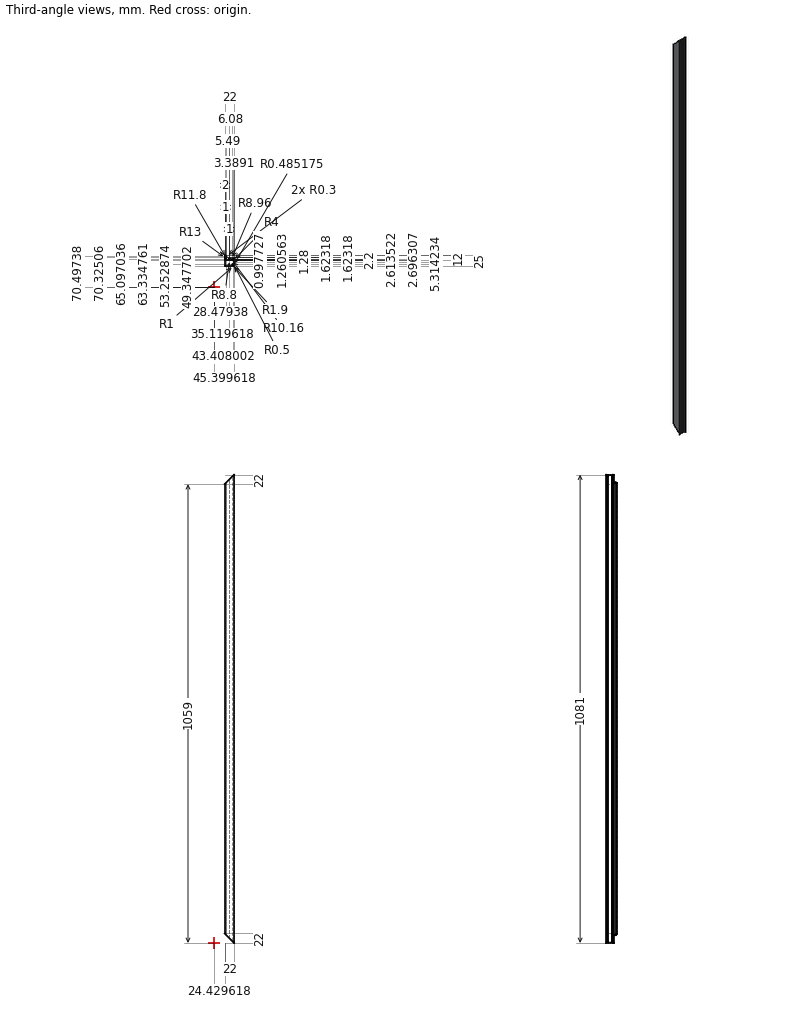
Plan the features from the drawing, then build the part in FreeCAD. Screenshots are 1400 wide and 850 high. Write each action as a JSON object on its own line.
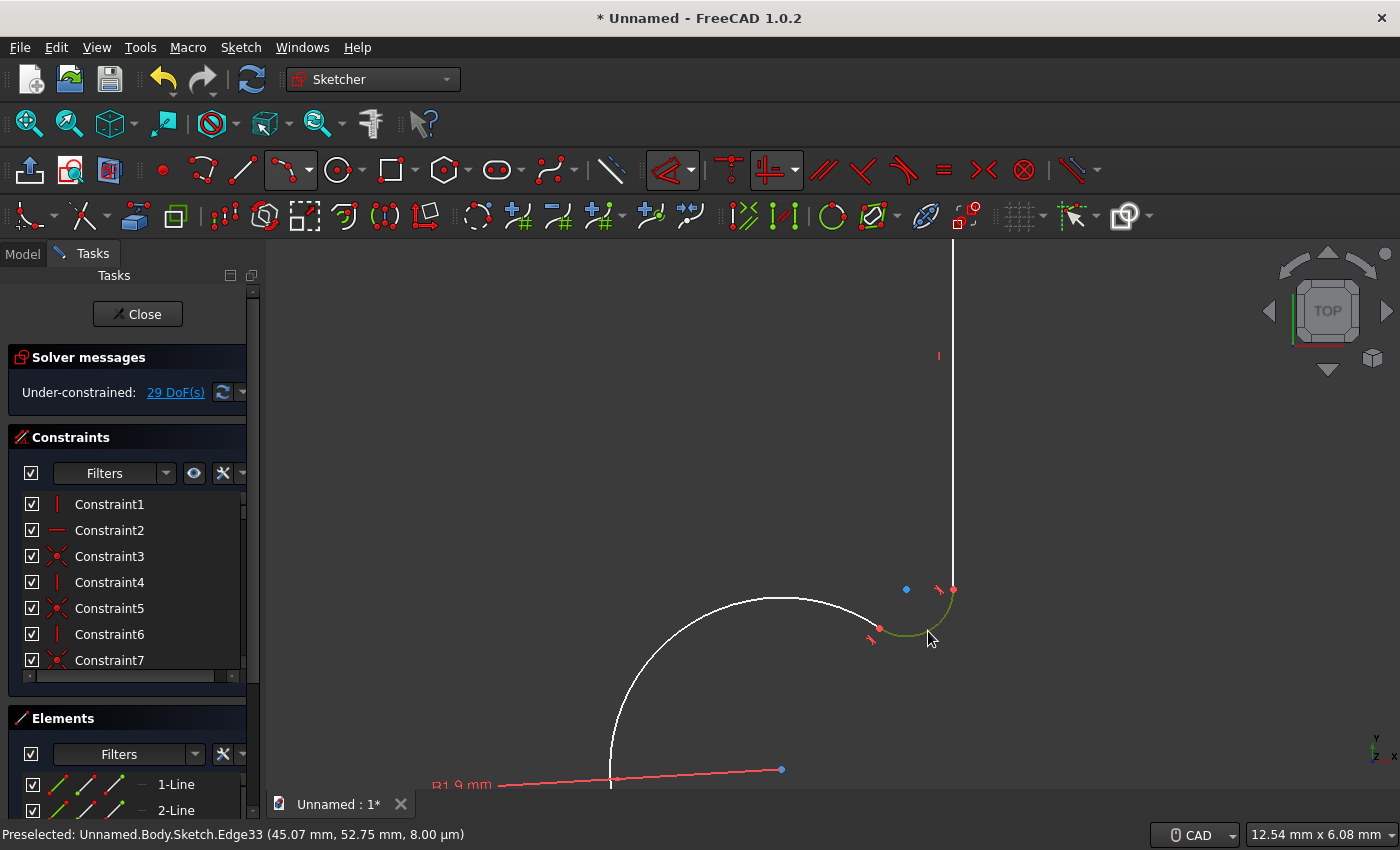
{"action": "key", "text": "k r"}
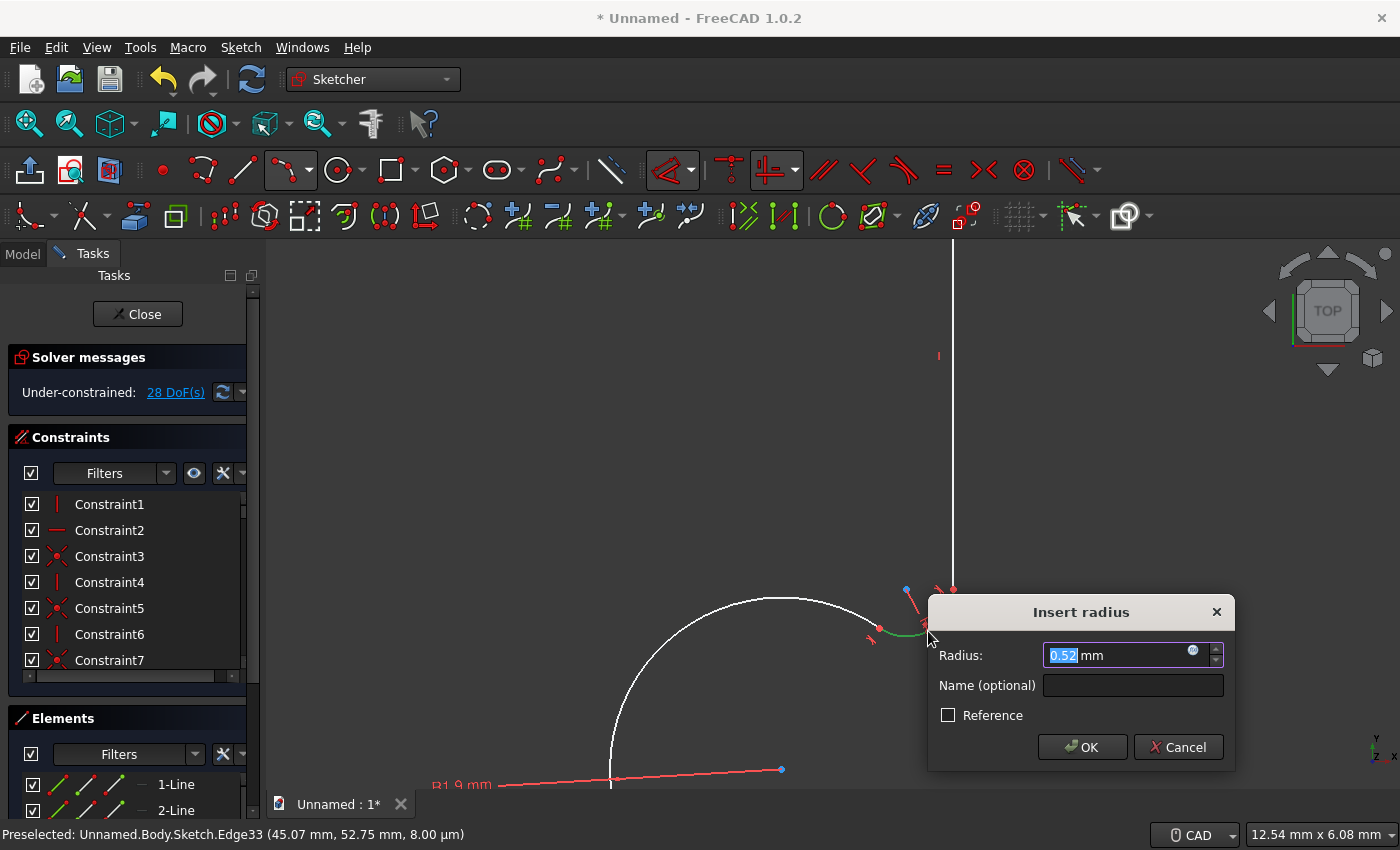
{"action": "type", "text": "0.5"}
{"action": "key", "text": "Return"}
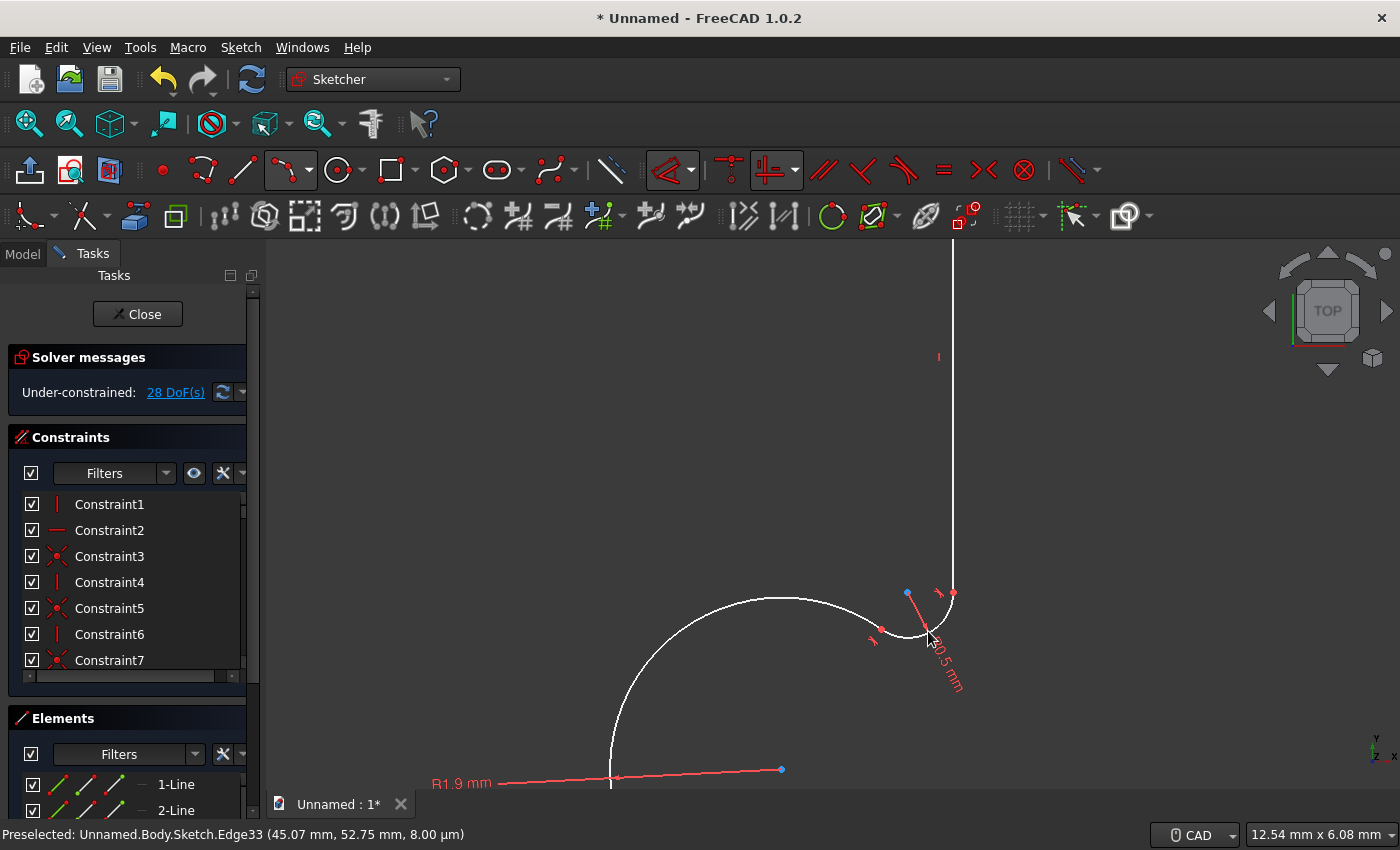
{"action": "scroll", "coordinate": [906, 633], "scroll_direction": "down", "scroll_amount": 9}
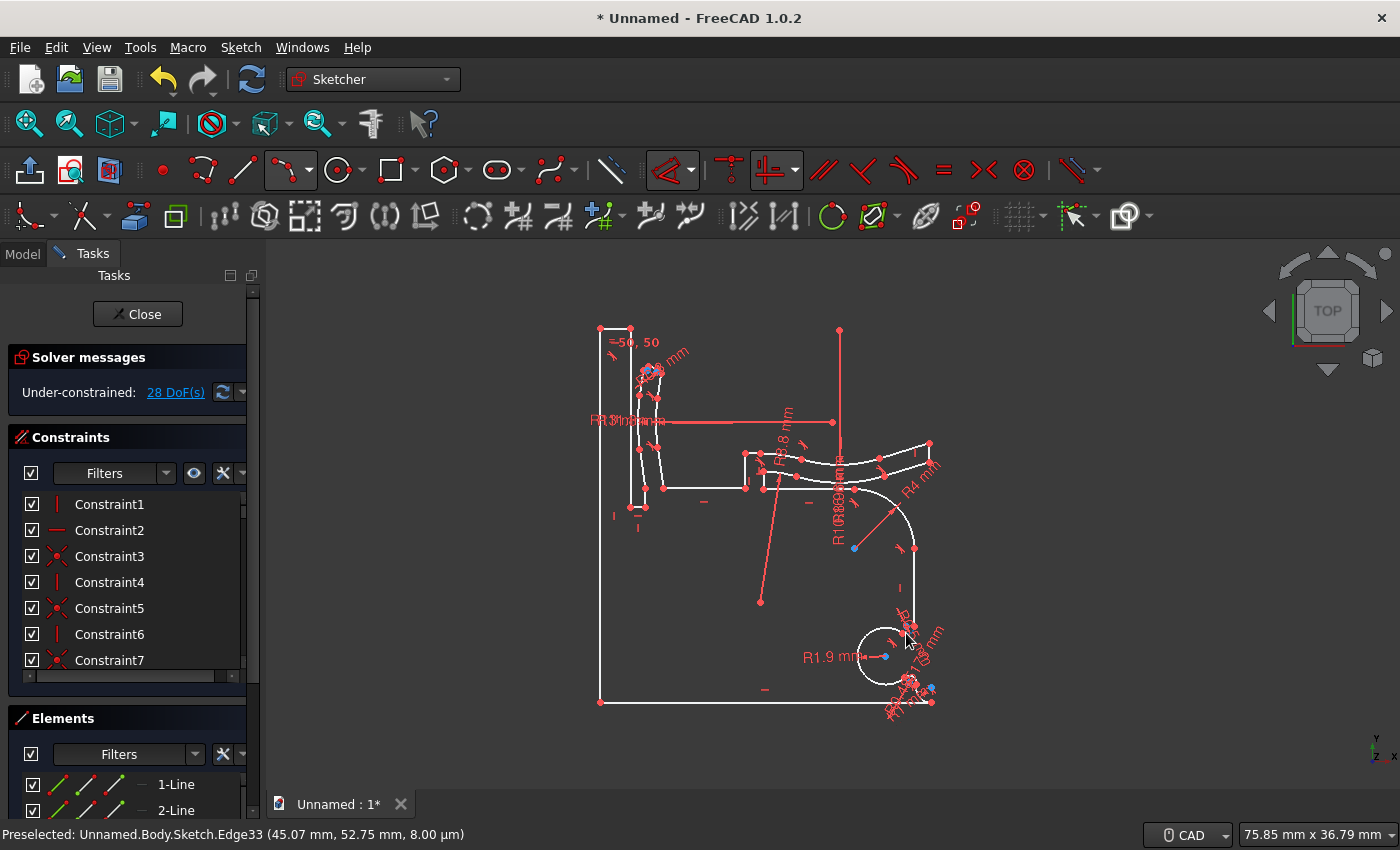
{"action": "scroll", "coordinate": [756, 453], "scroll_direction": "up", "scroll_amount": 6}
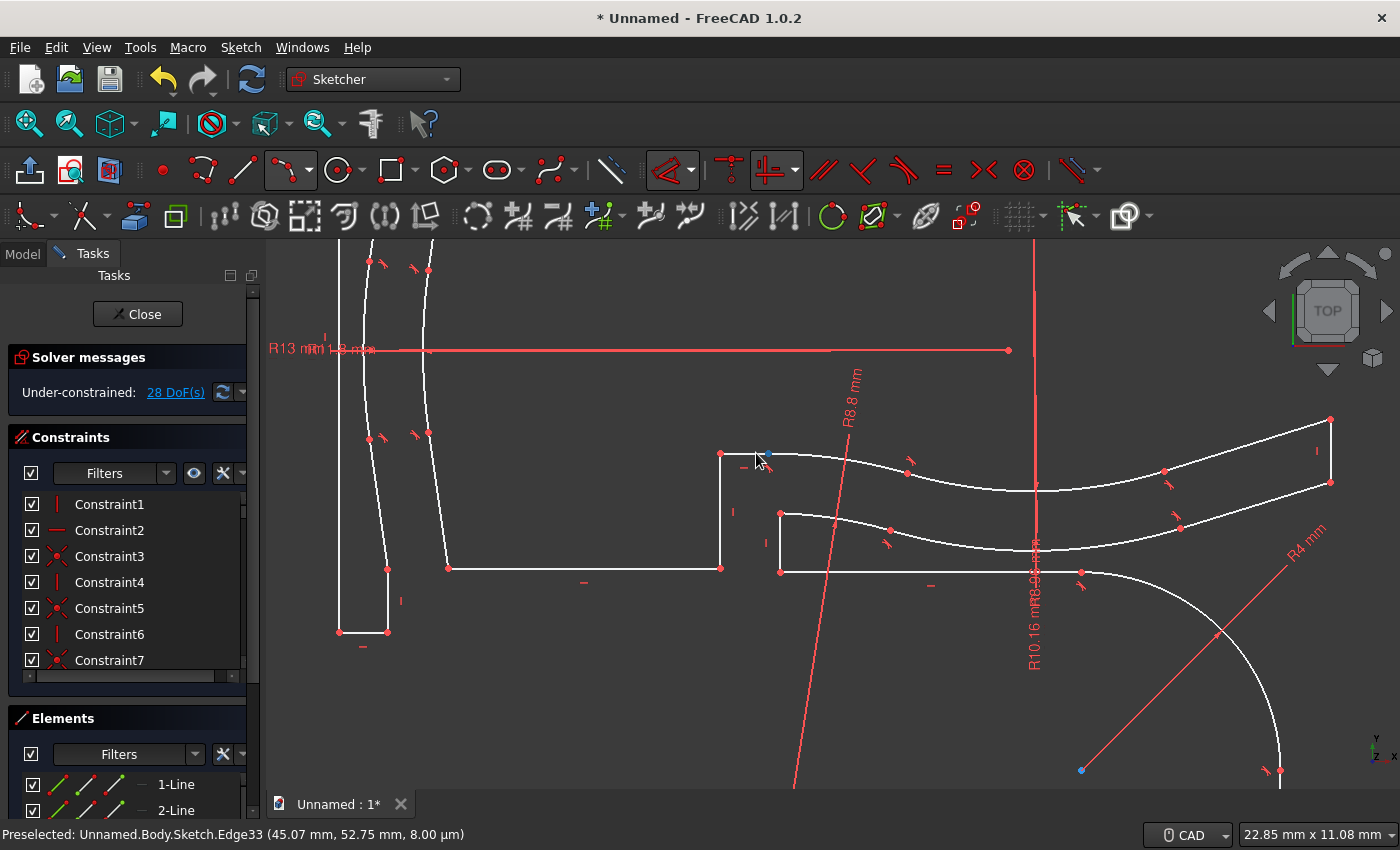
{"action": "left_click", "coordinate": [754, 454]}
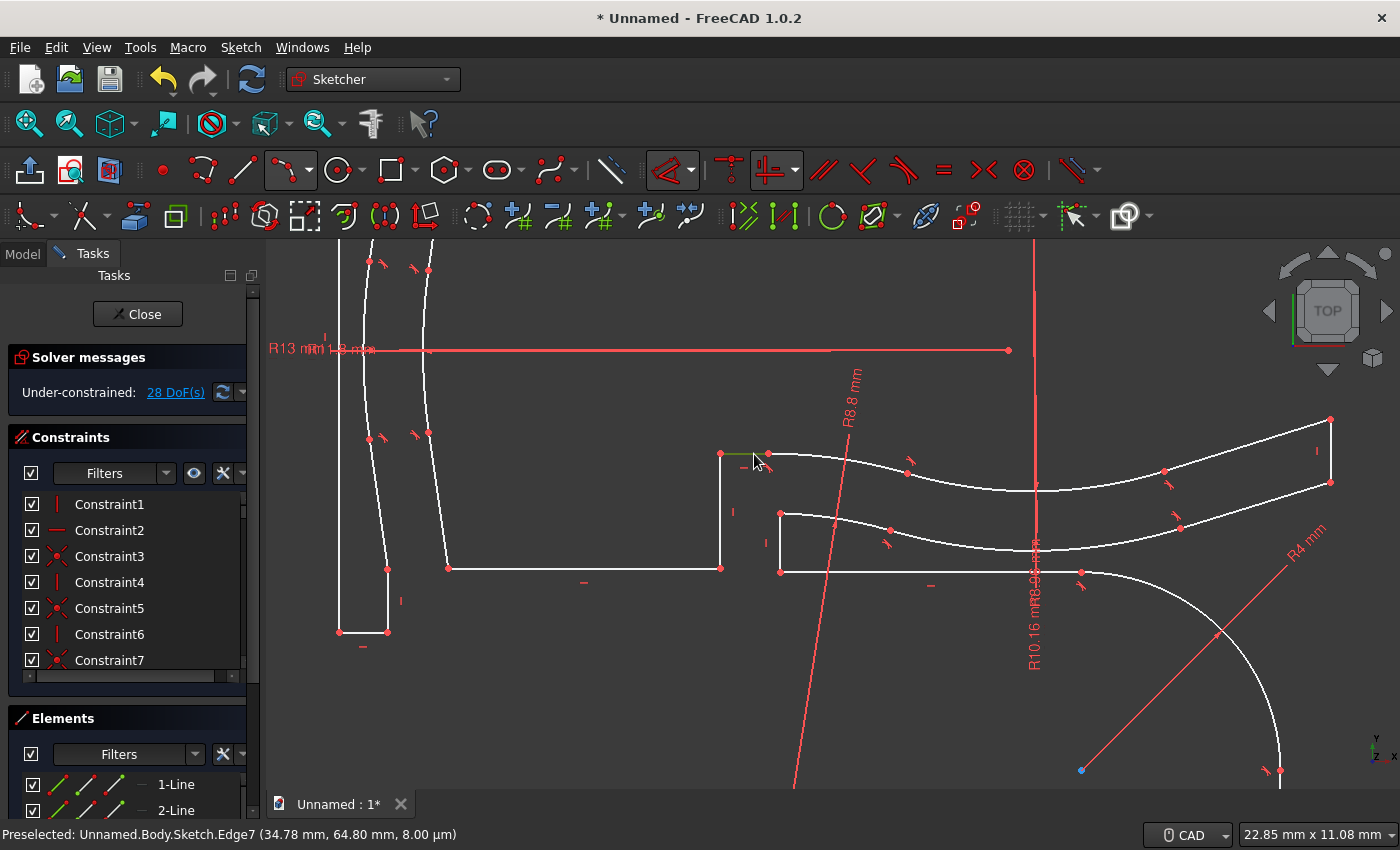
{"action": "left_click", "coordinate": [694, 170]}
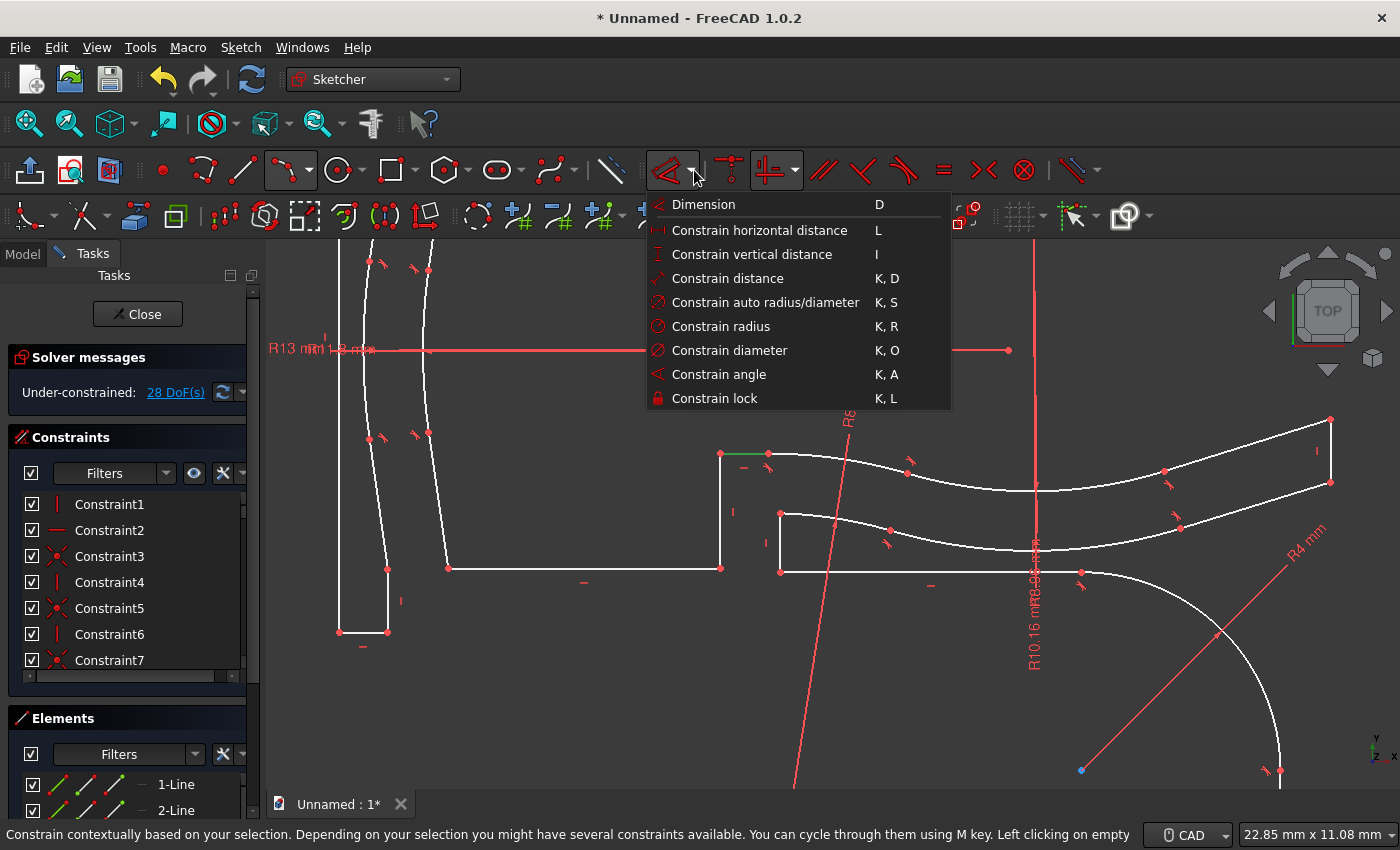
{"action": "left_click", "coordinate": [799, 230]}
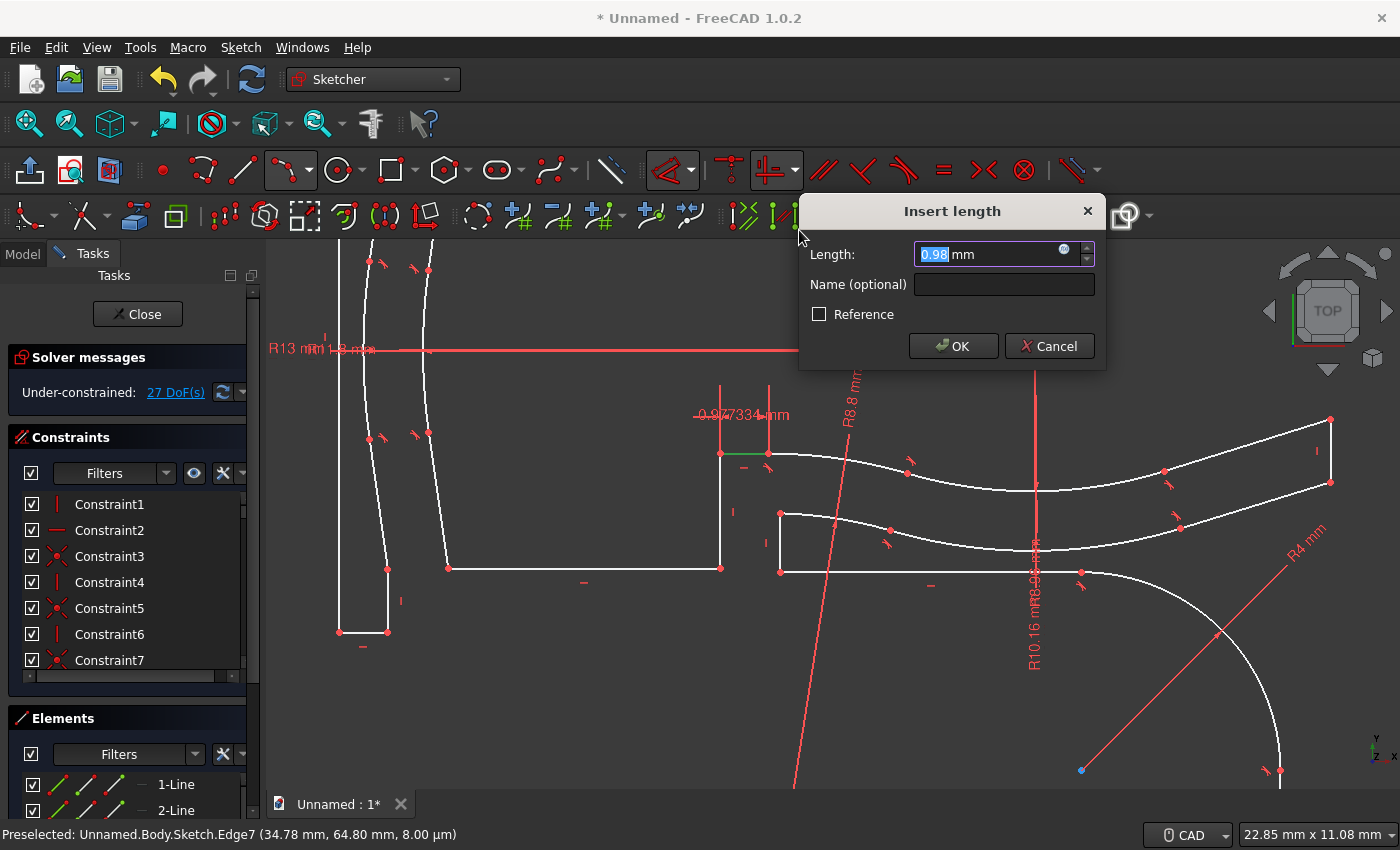
{"action": "type", "text": "1"}
{"action": "key", "text": "Return"}